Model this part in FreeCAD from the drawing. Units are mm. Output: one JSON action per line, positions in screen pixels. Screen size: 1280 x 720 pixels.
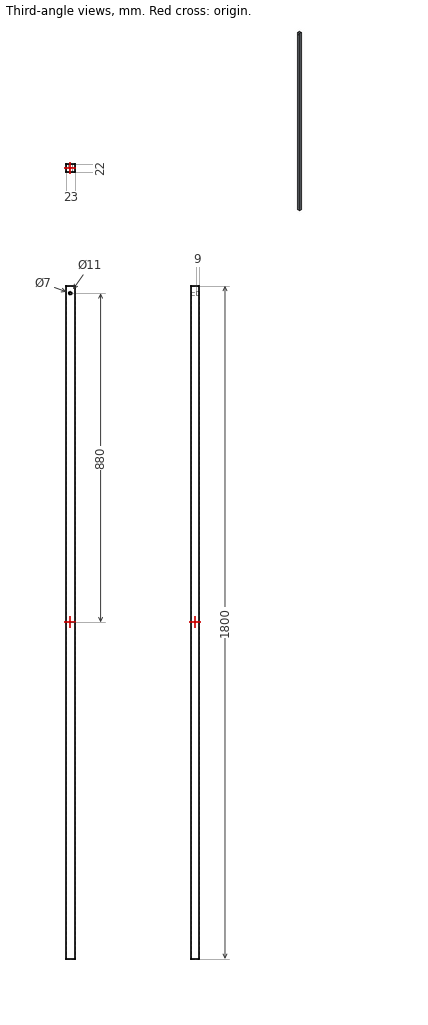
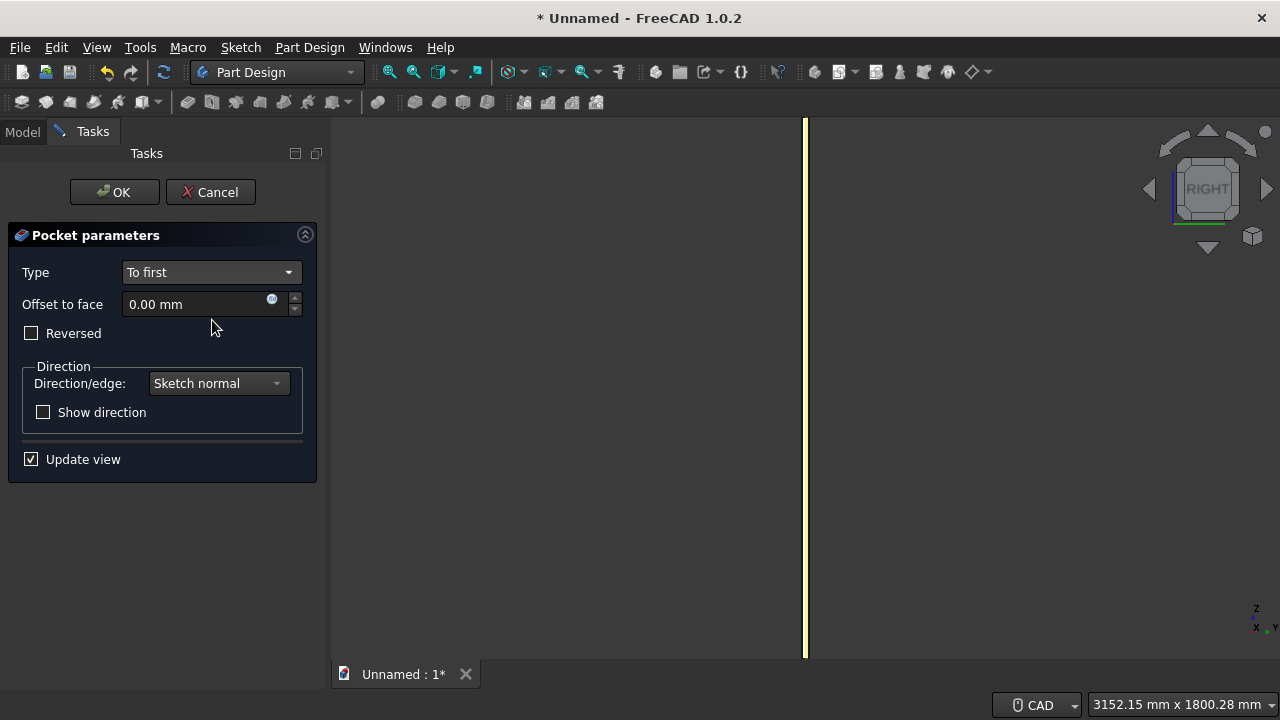
{"action": "left_click", "coordinate": [30, 333]}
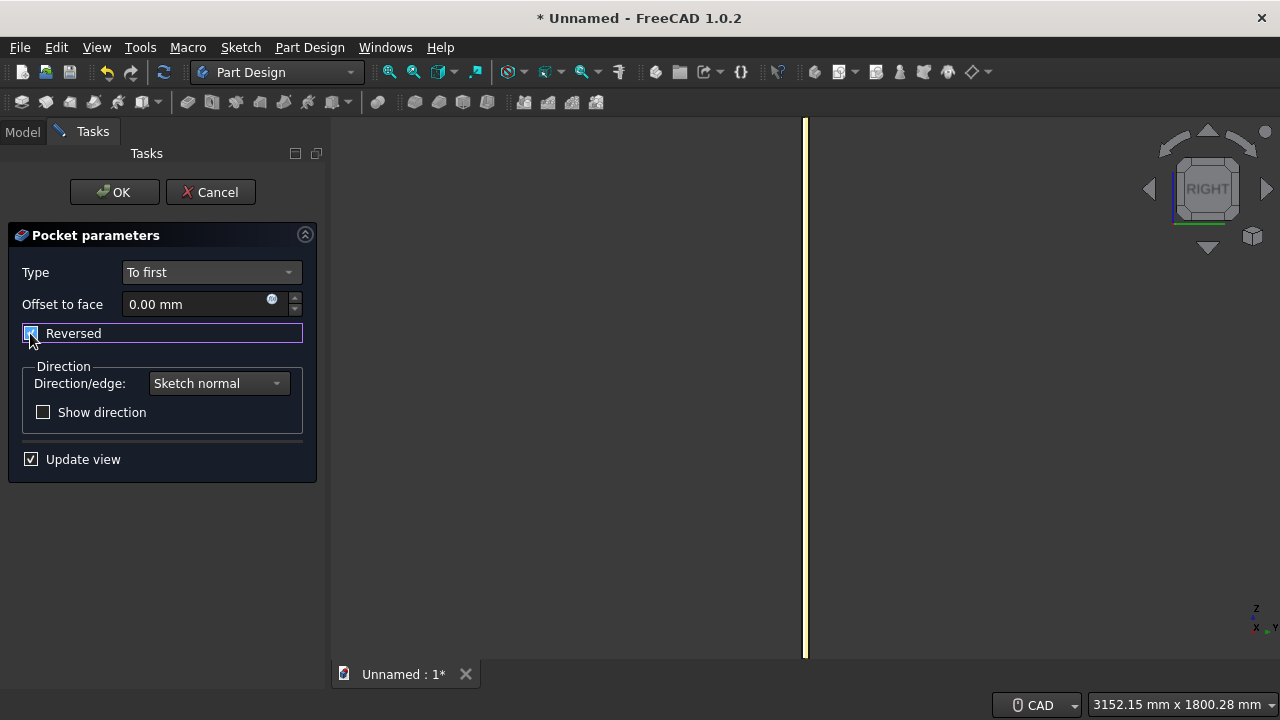
{"action": "left_click", "coordinate": [115, 192]}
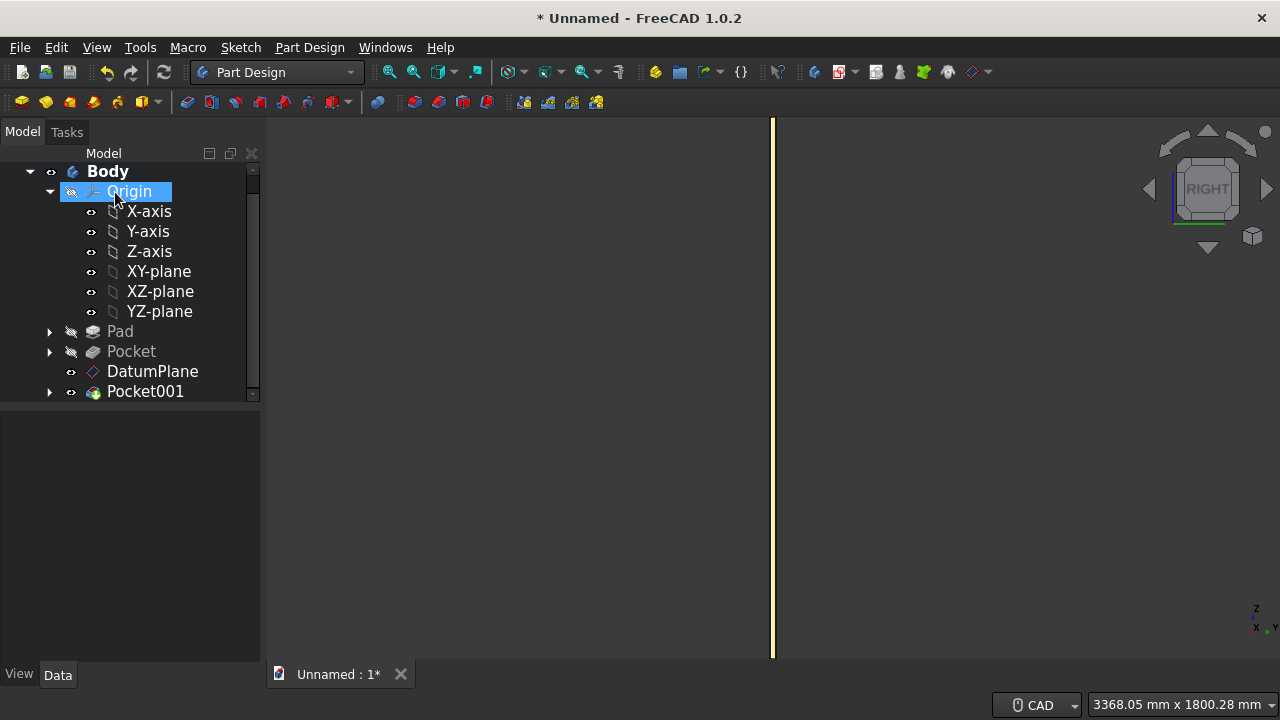
{"action": "left_click", "coordinate": [116, 372]}
{"action": "key", "text": "space"}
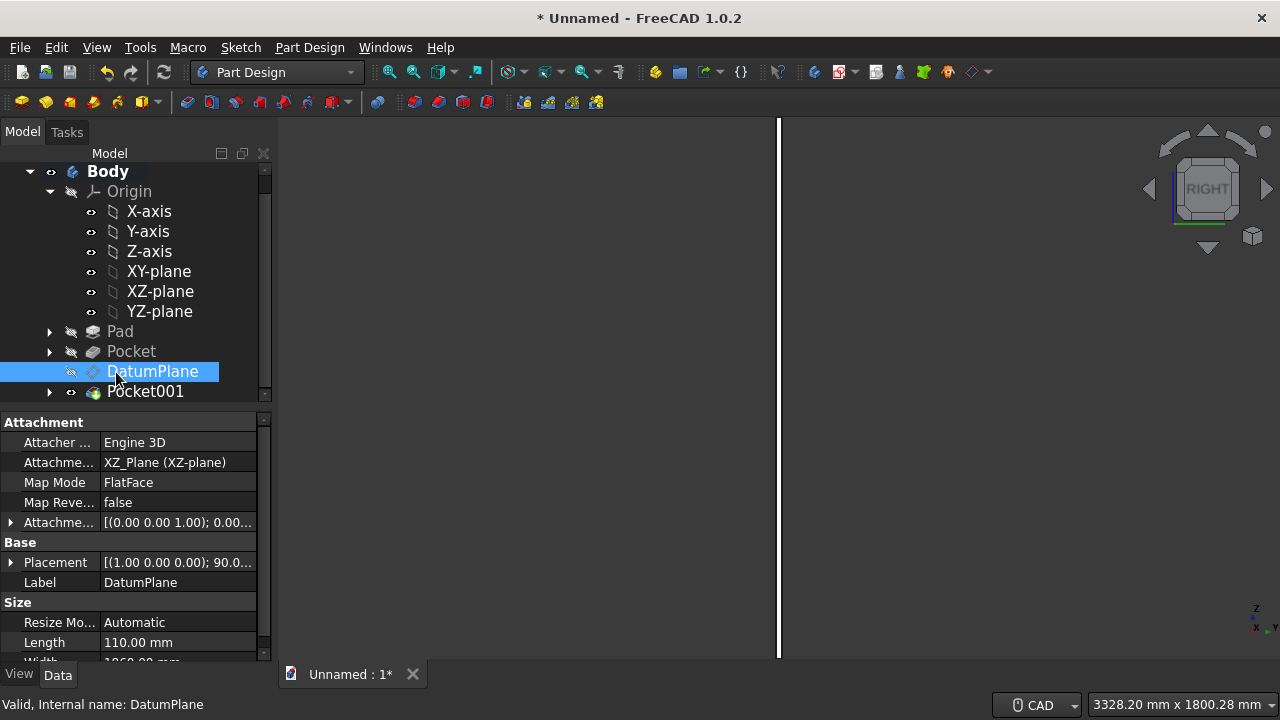
{"action": "key", "text": "0"}